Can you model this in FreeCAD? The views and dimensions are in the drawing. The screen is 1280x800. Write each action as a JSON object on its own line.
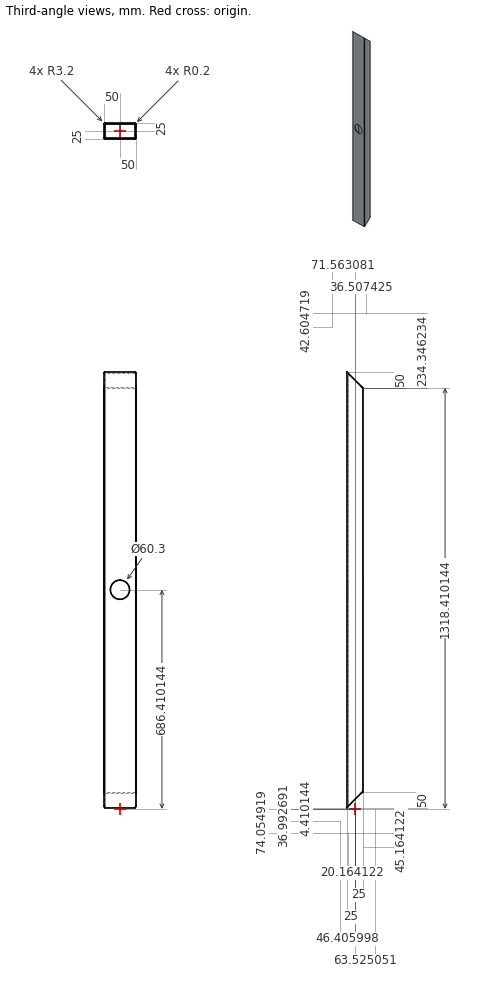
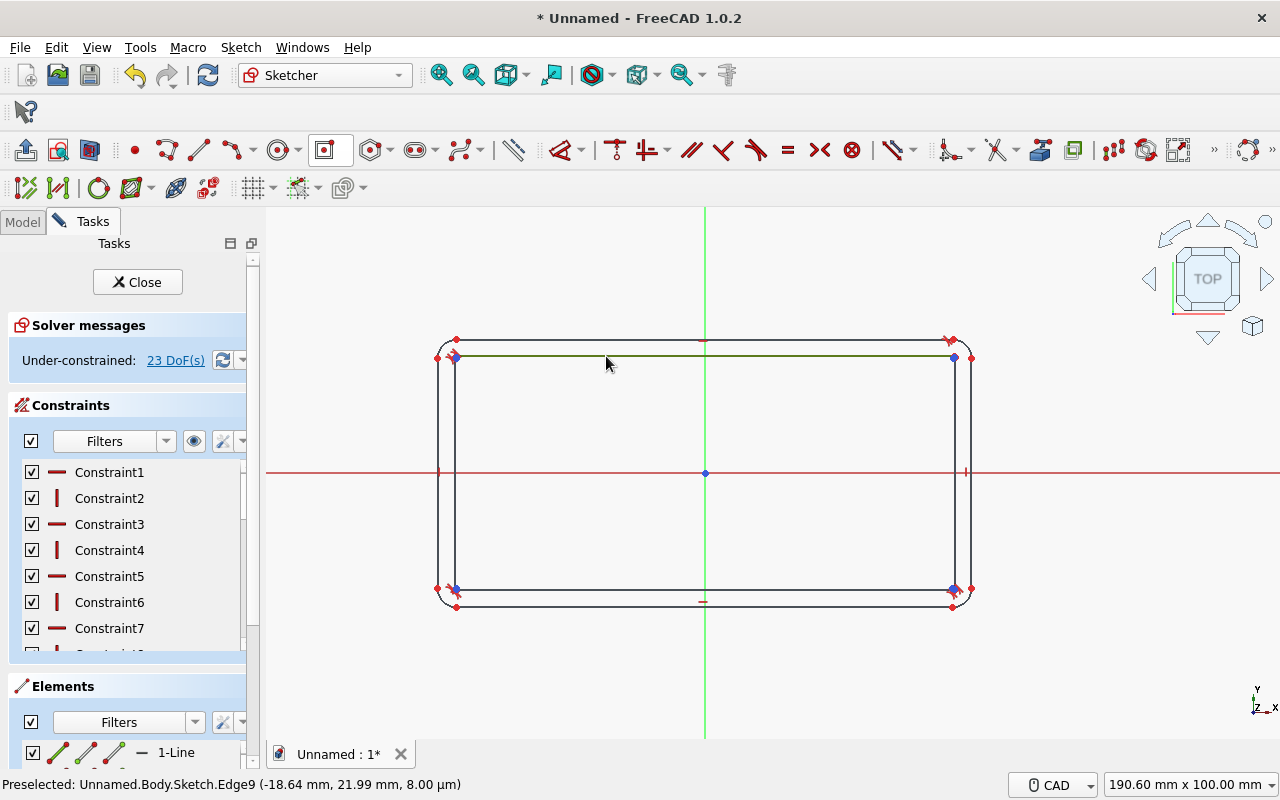
{"action": "scroll", "coordinate": [455, 357], "scroll_direction": "up", "scroll_amount": 14}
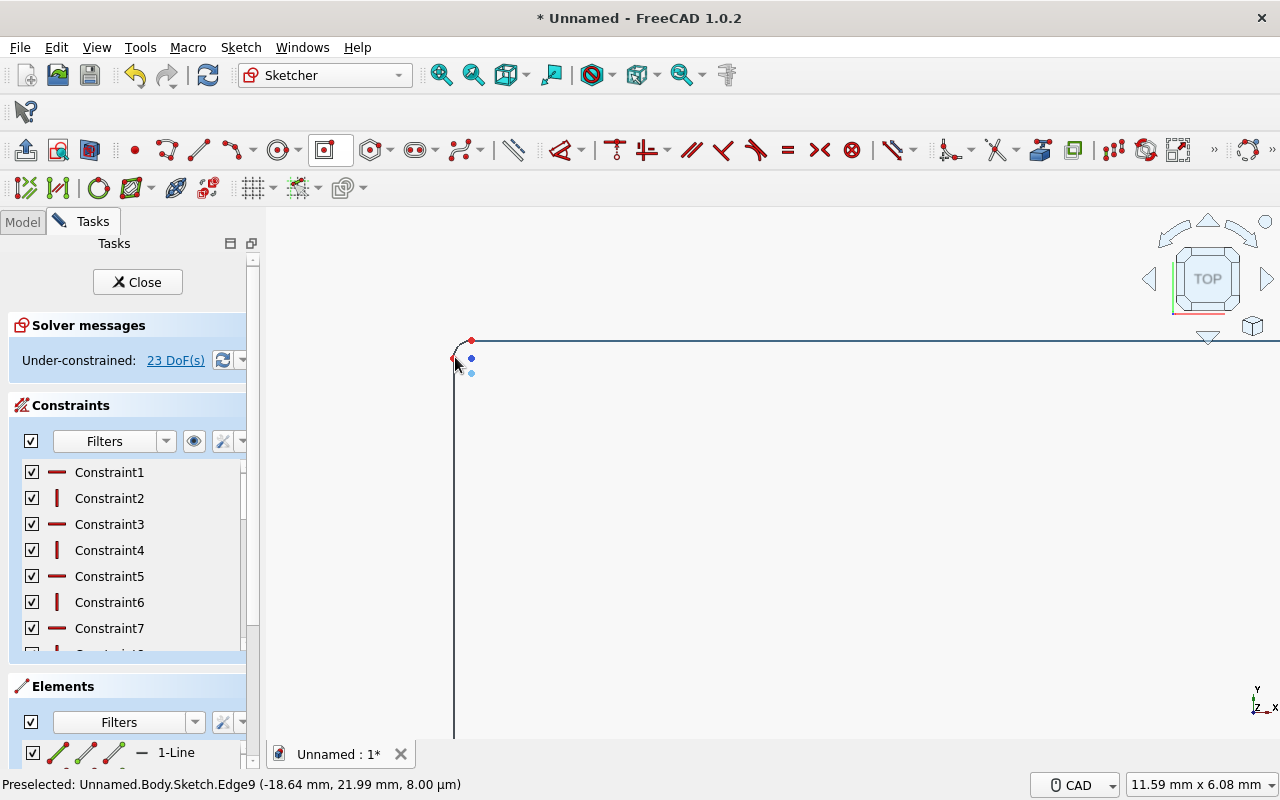
{"action": "left_click", "coordinate": [459, 346]}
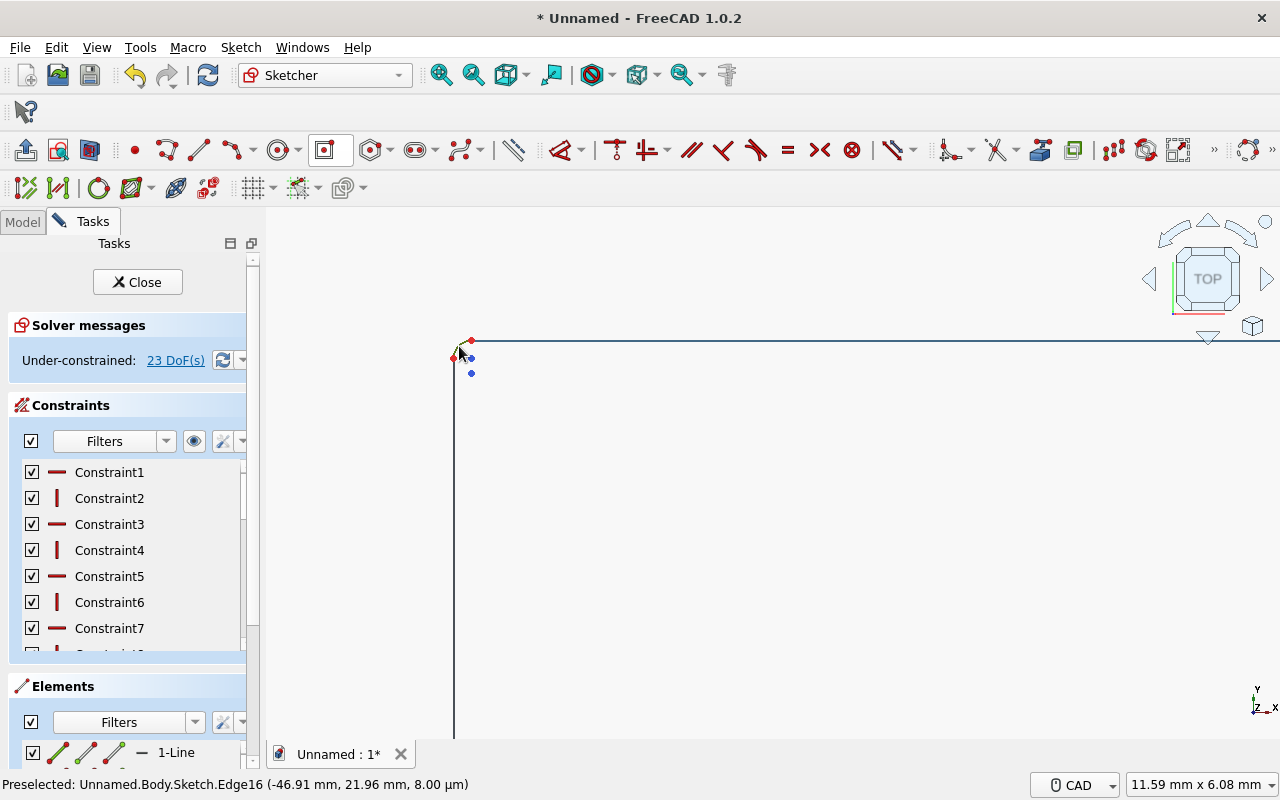
{"action": "key", "text": "t"}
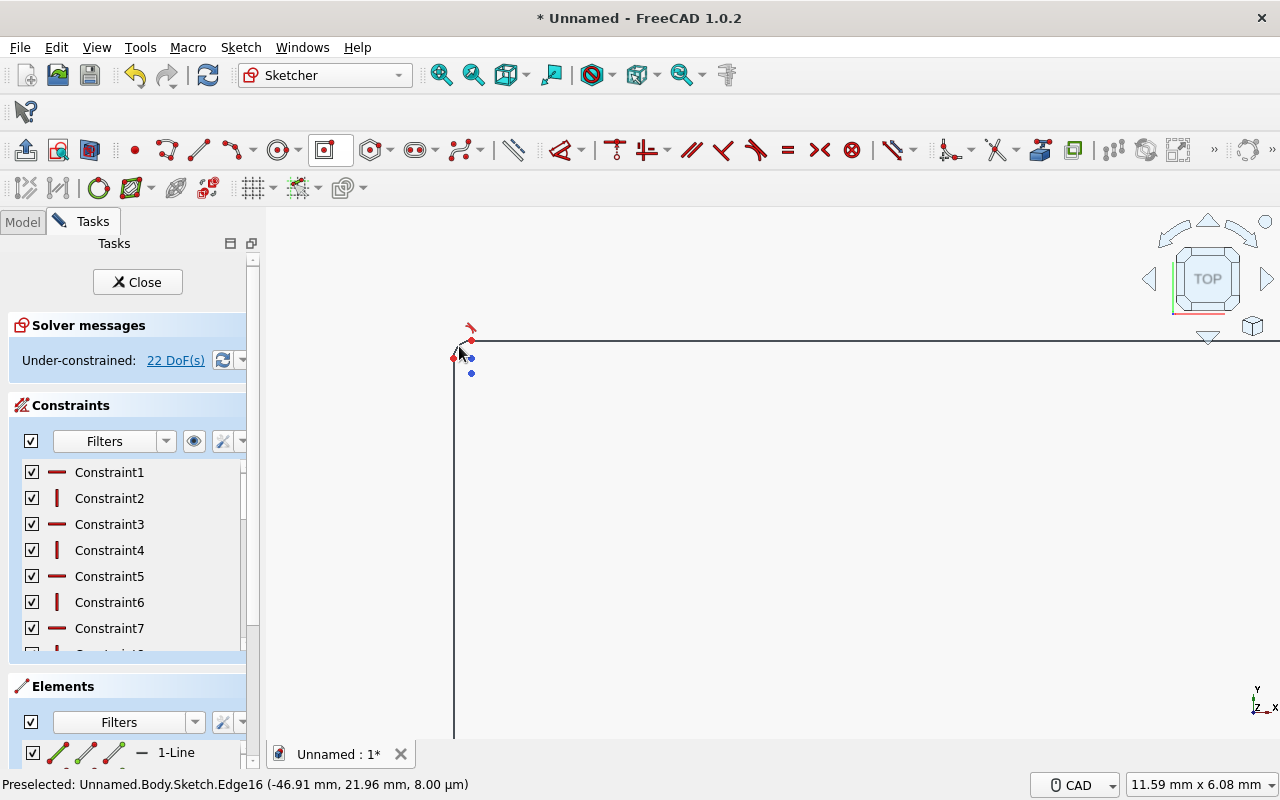
{"action": "scroll", "coordinate": [454, 357], "scroll_direction": "down", "scroll_amount": 14}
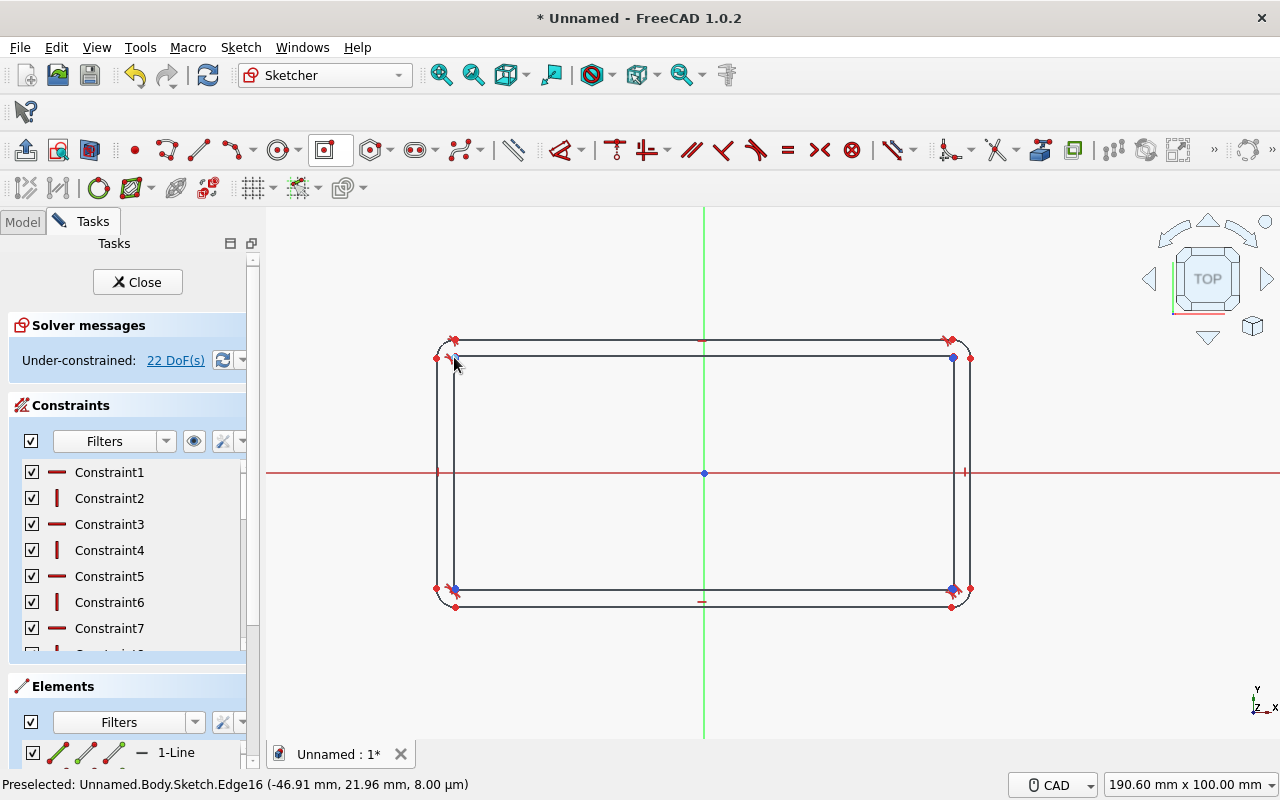
{"action": "left_click", "coordinate": [954, 427]}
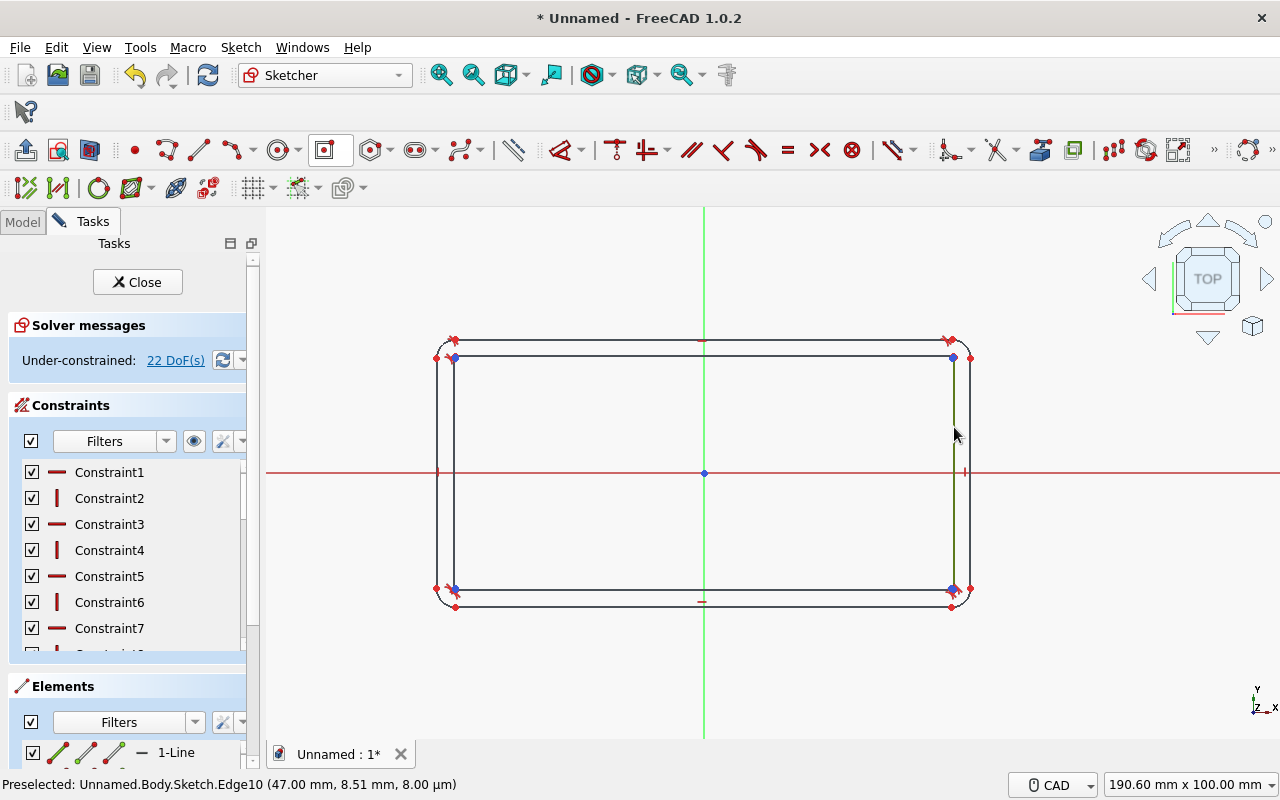
{"action": "scroll", "coordinate": [954, 357], "scroll_direction": "up", "scroll_amount": 14}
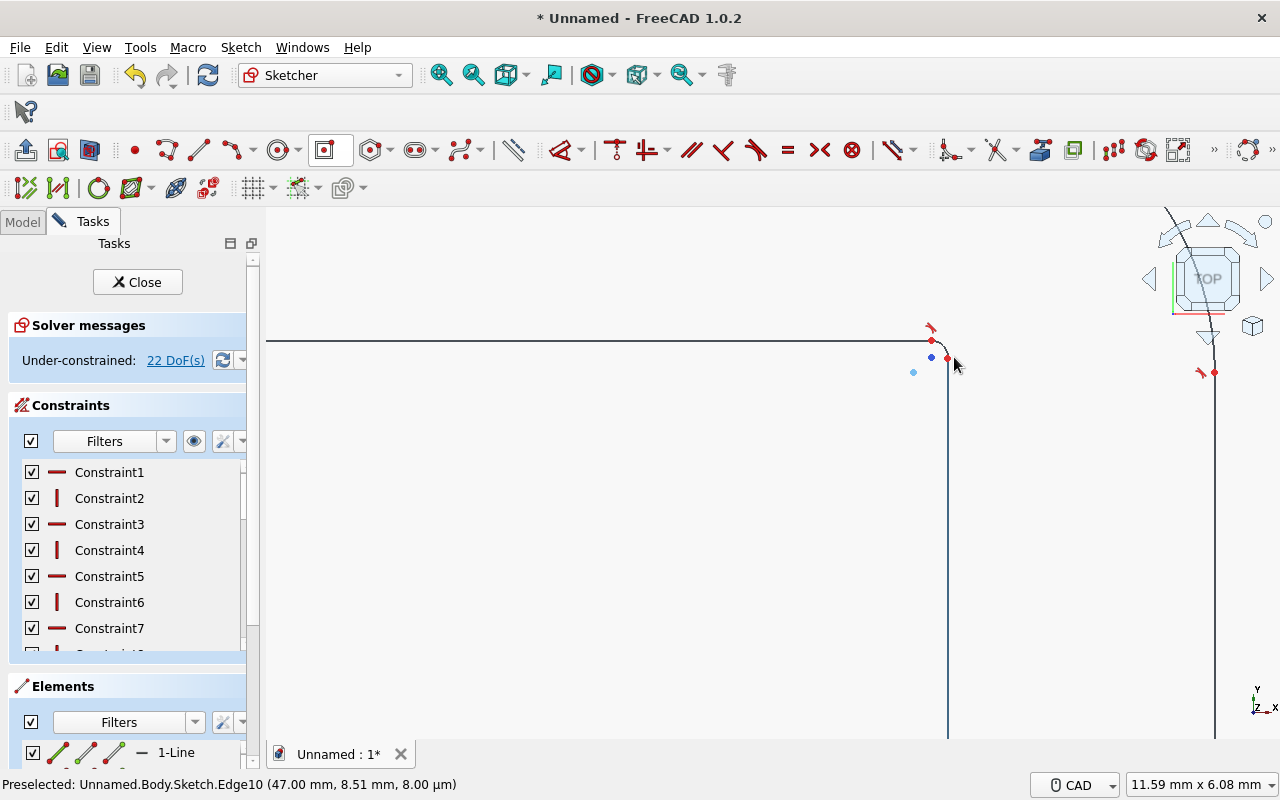
{"action": "left_click", "coordinate": [944, 346]}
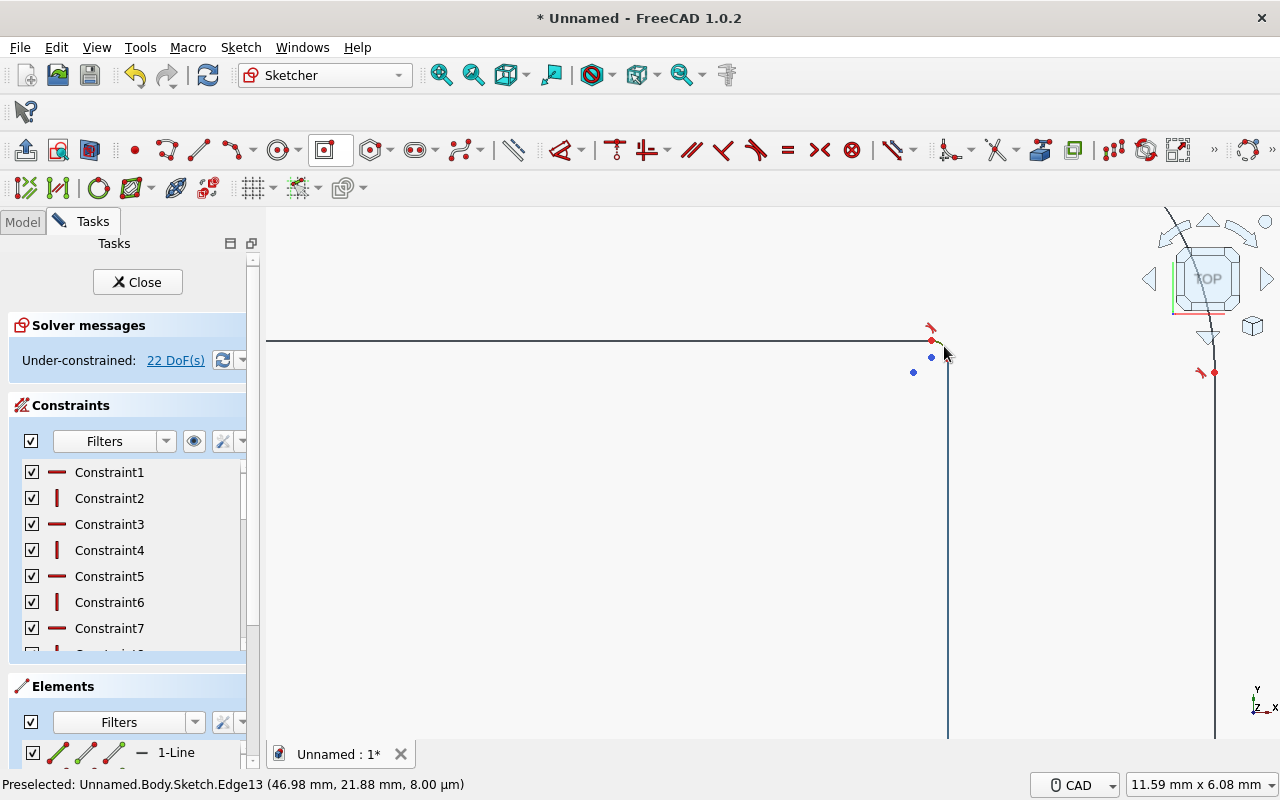
{"action": "left_click", "coordinate": [756, 150]}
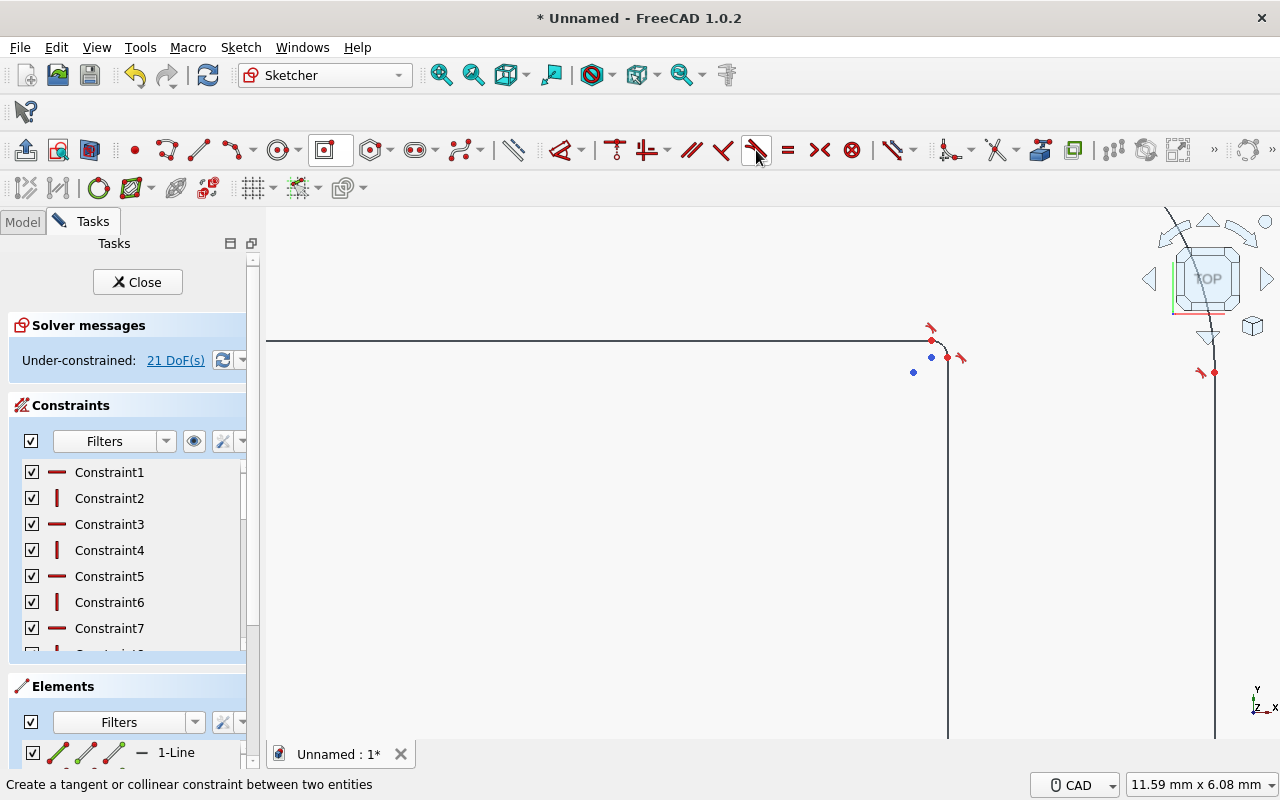
{"action": "scroll", "coordinate": [955, 357], "scroll_direction": "down", "scroll_amount": 14}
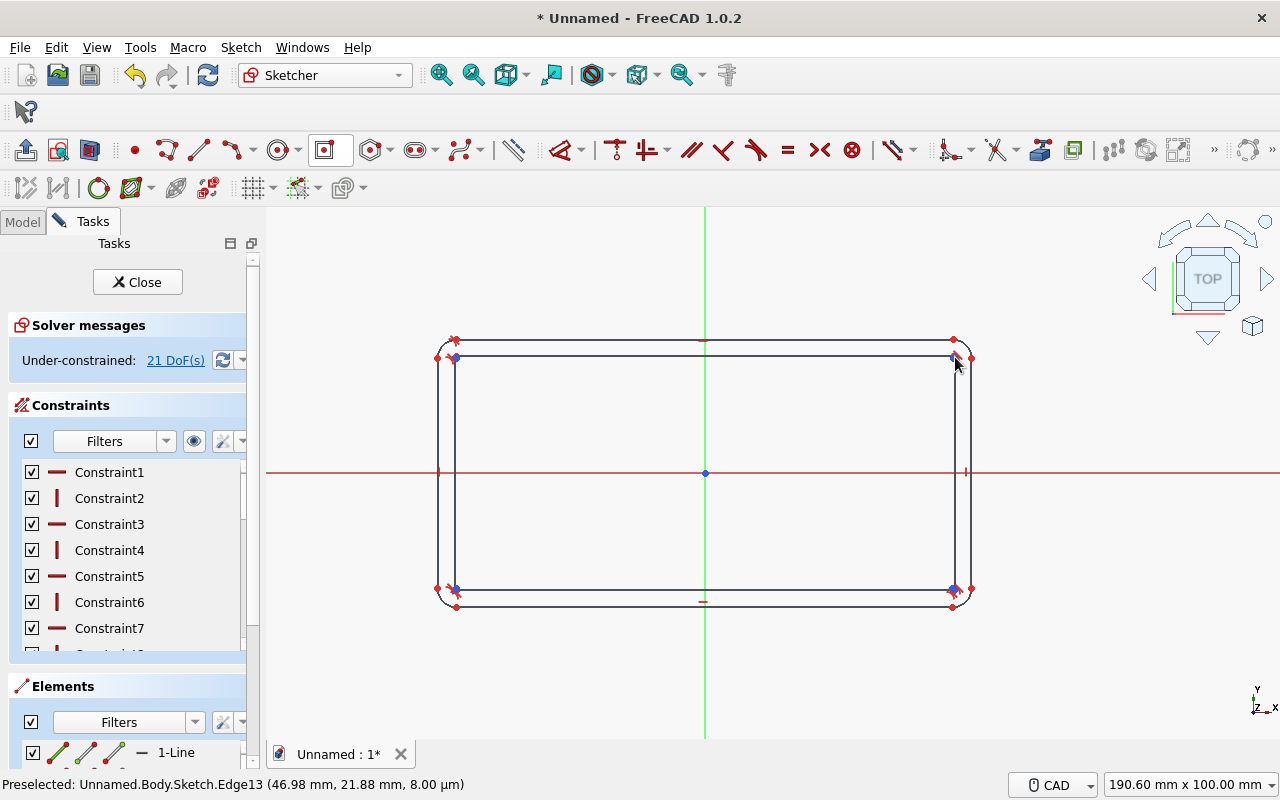
{"action": "left_click", "coordinate": [955, 427]}